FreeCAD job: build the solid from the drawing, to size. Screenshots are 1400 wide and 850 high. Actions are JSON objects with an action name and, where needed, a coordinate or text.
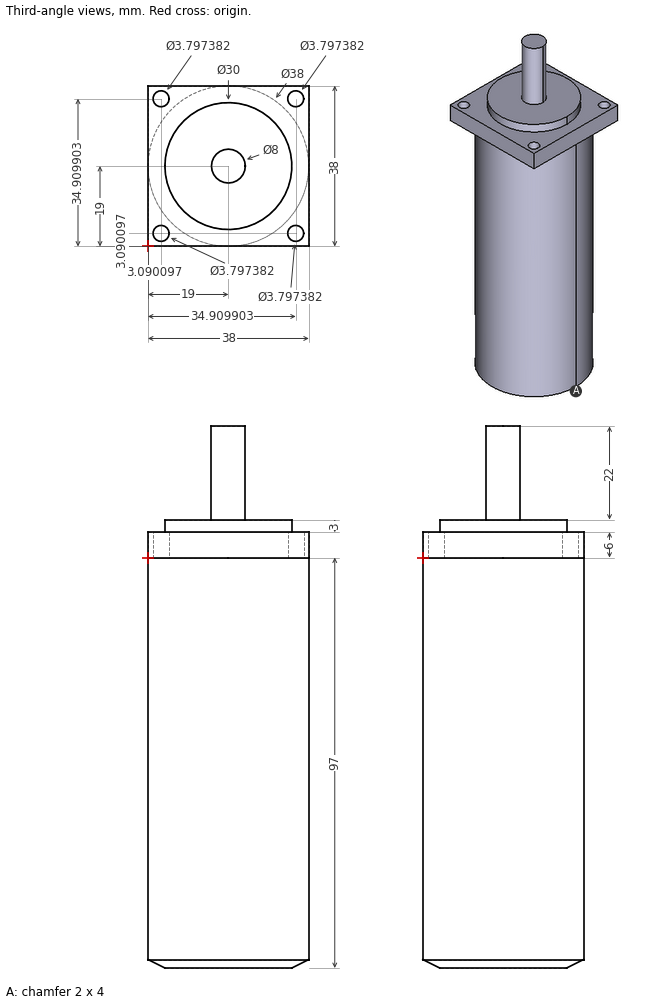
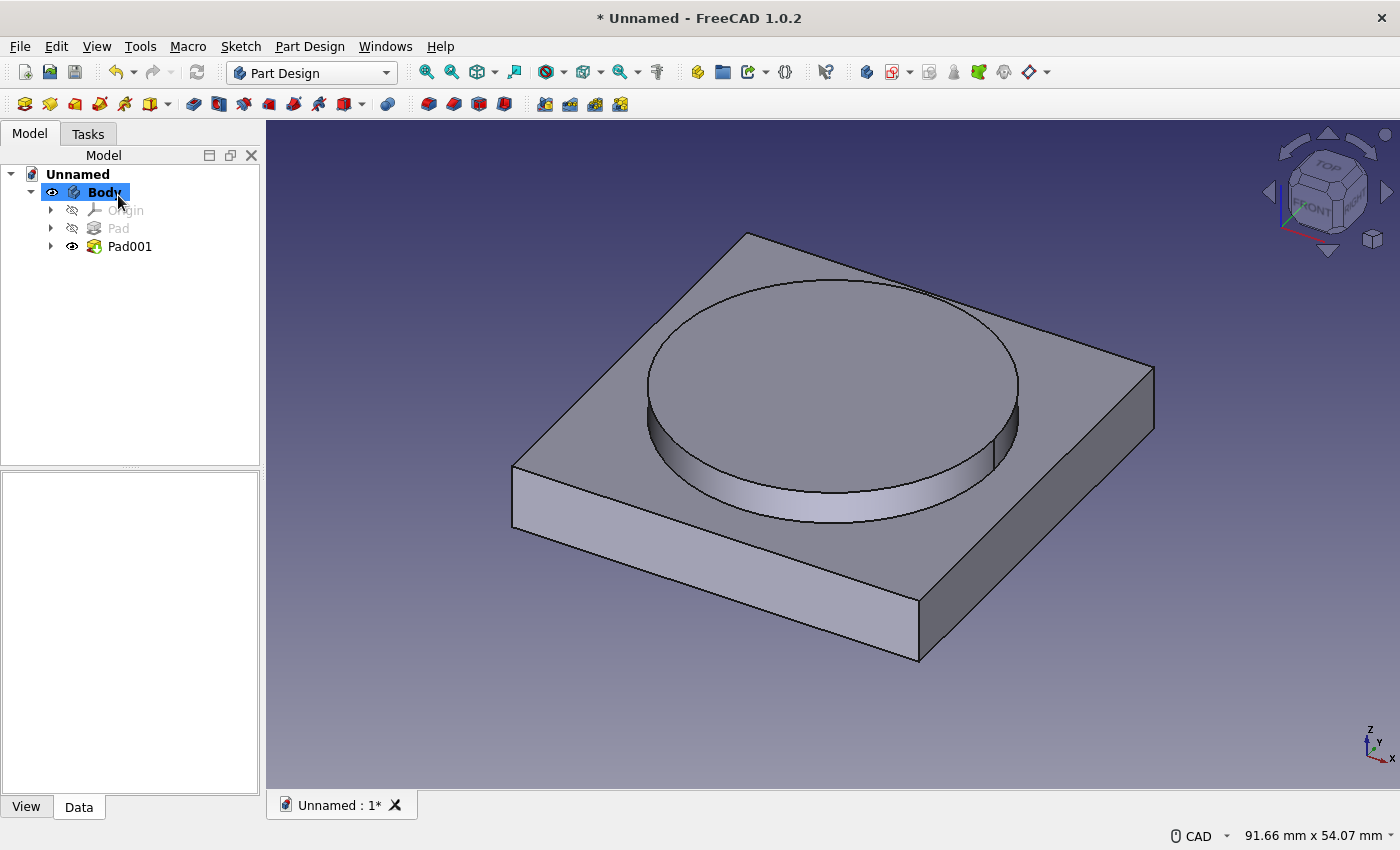
{"action": "left_click", "coordinate": [833, 385]}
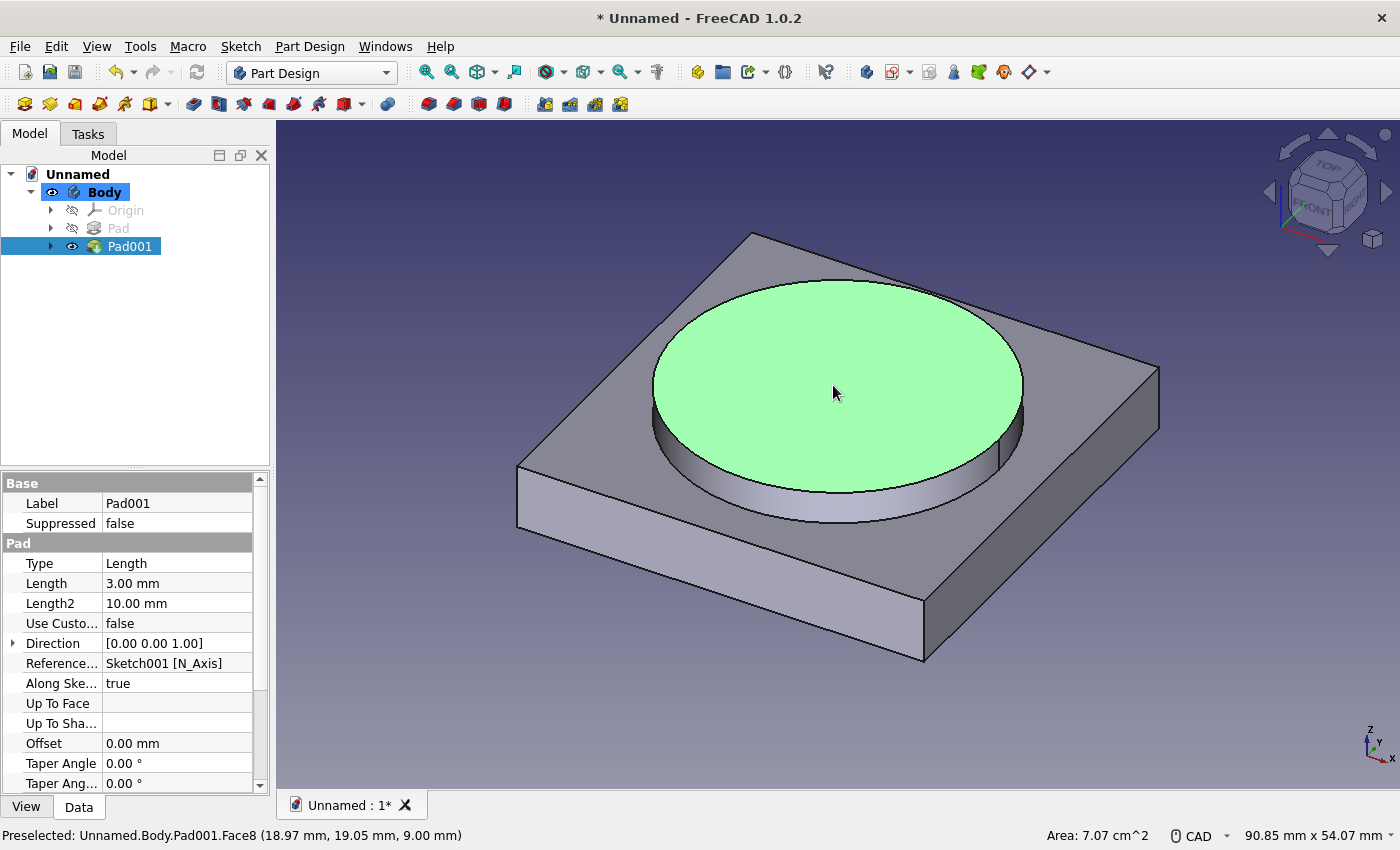
{"action": "left_click", "coordinate": [892, 72]}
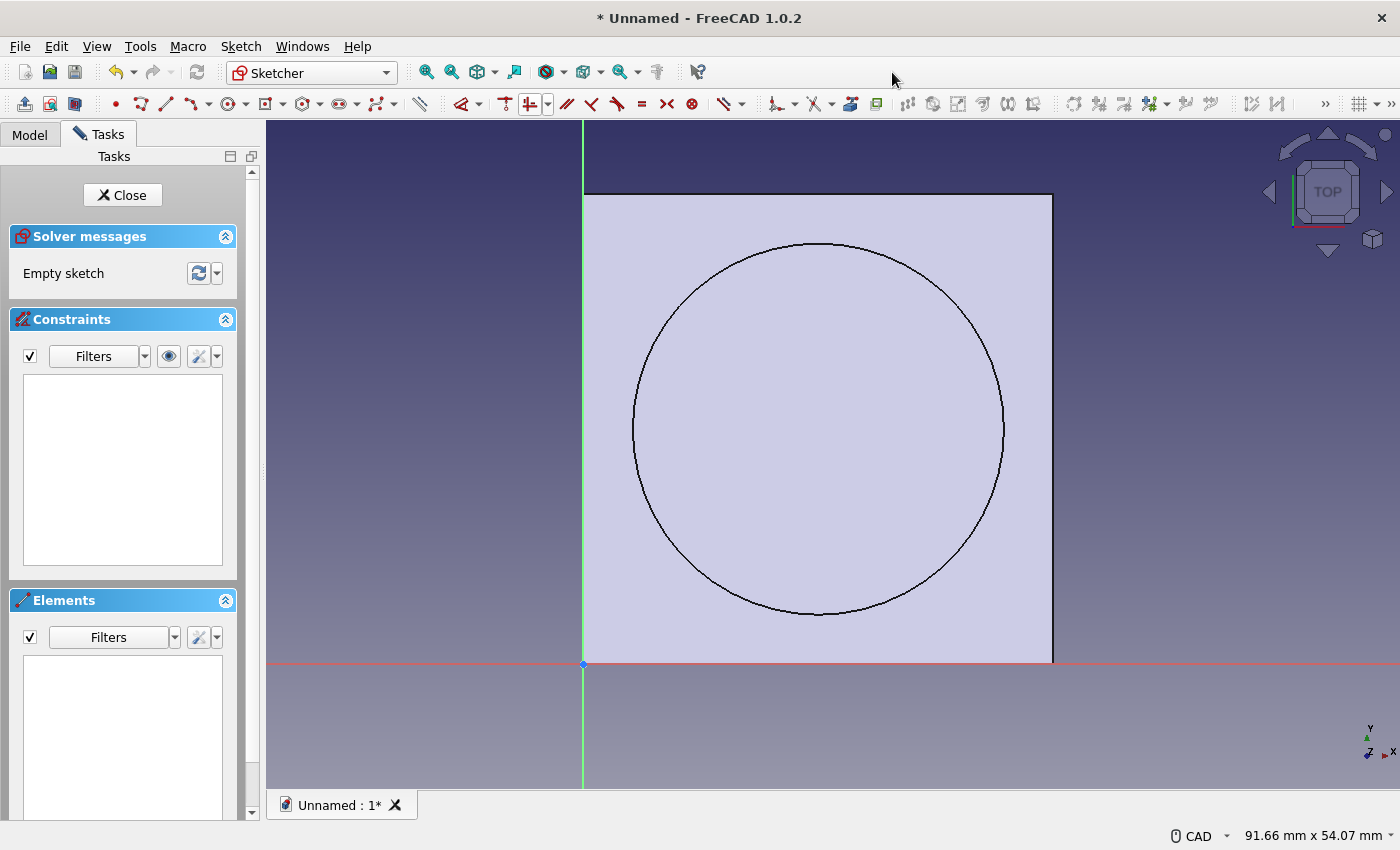
{"action": "scroll", "coordinate": [836, 421], "scroll_direction": "up", "scroll_amount": 7}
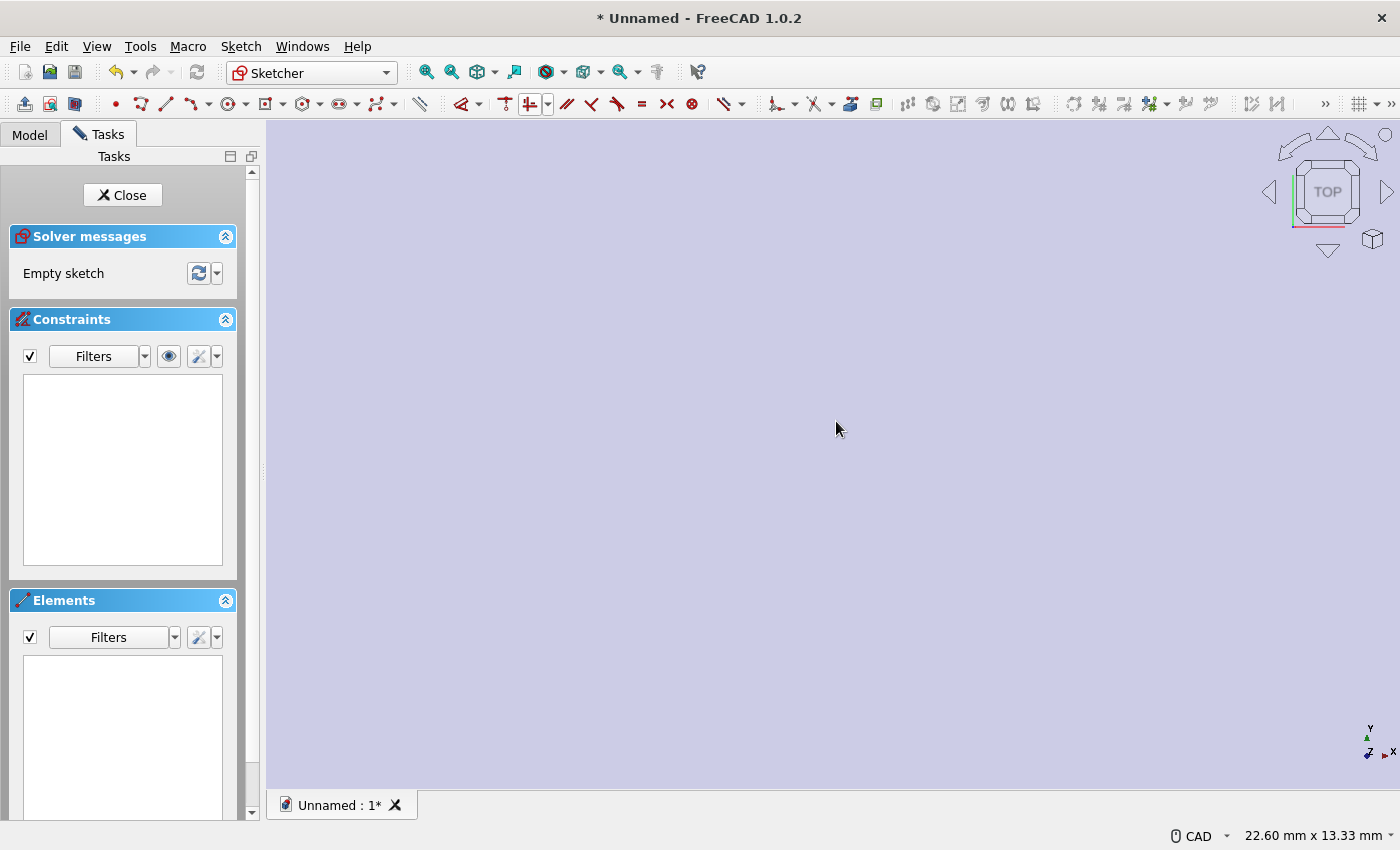
{"action": "left_click", "coordinate": [228, 104]}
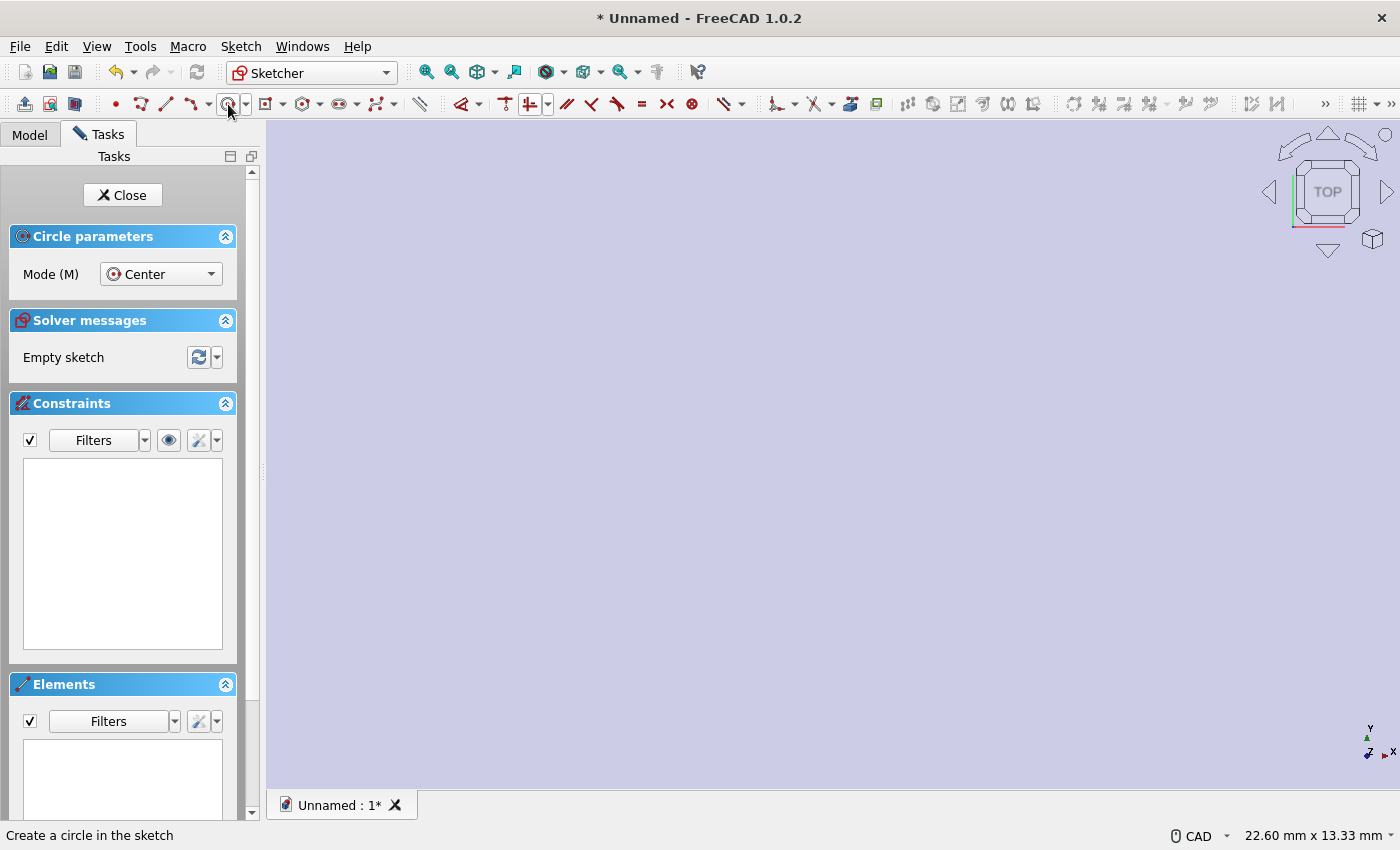
{"action": "left_click", "coordinate": [763, 453]}
{"action": "mouse_move", "coordinate": [905, 311]}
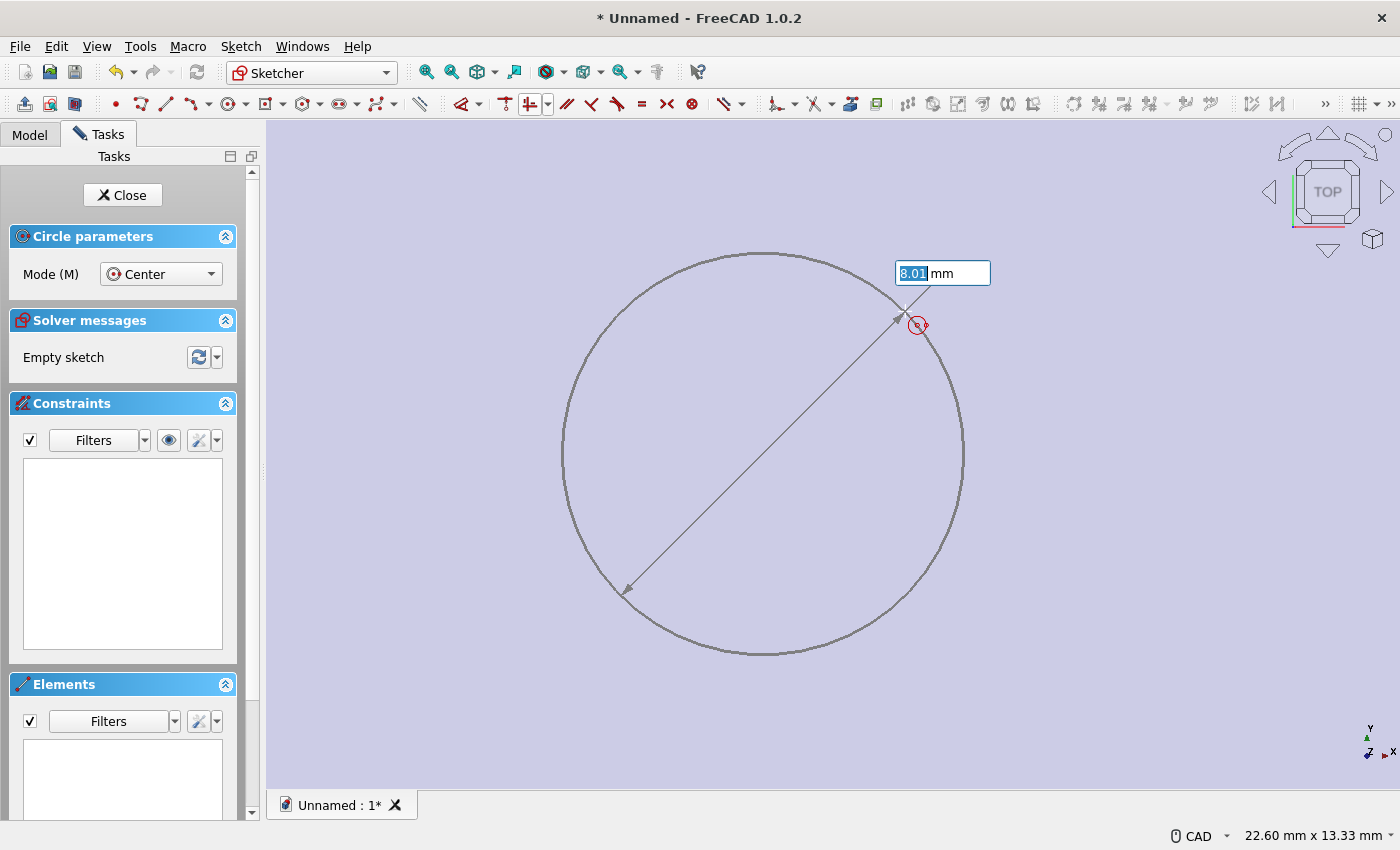
{"action": "type", "text": "8"}
{"action": "key", "text": "Return"}
{"action": "key", "text": "Escape"}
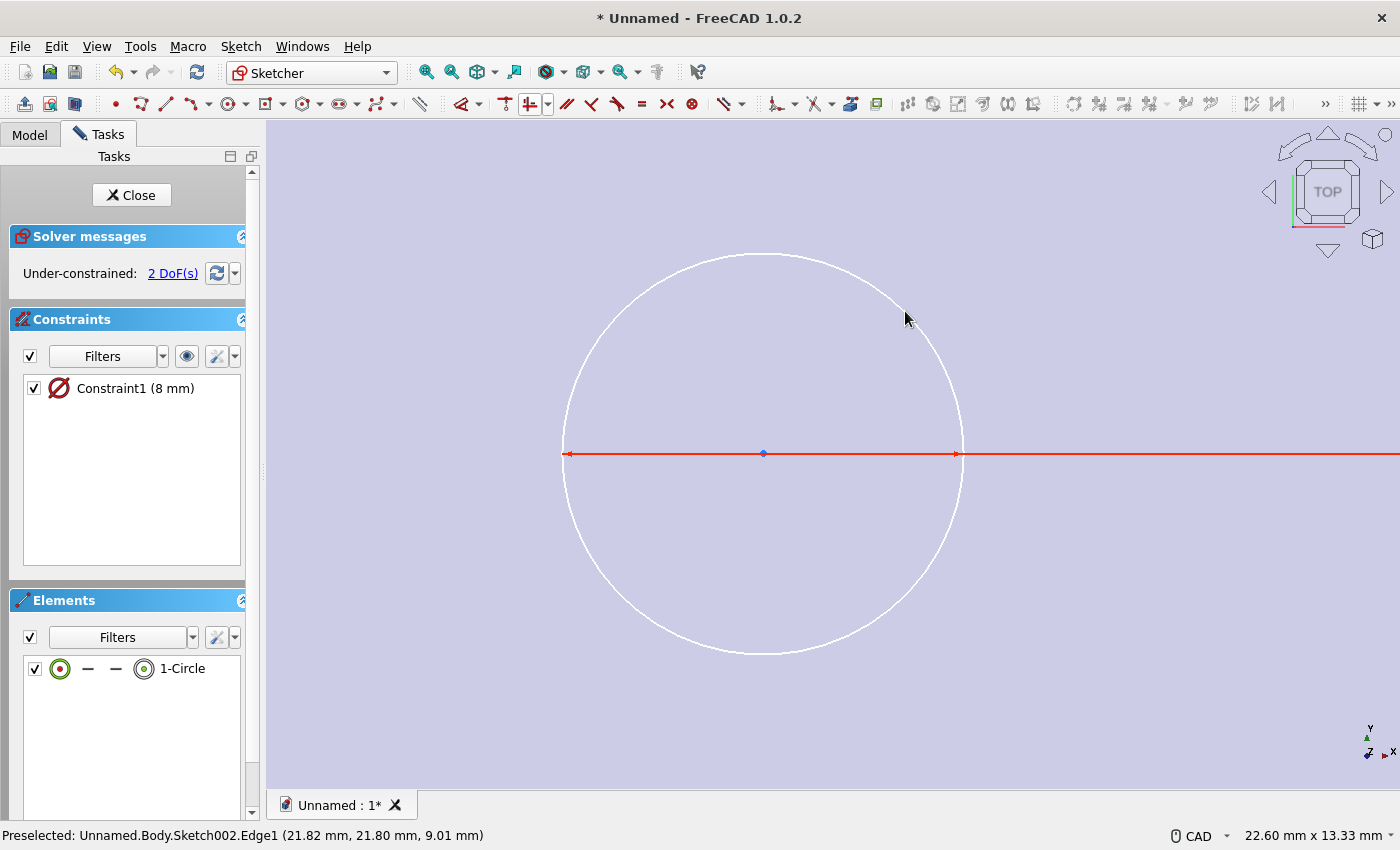
{"action": "key", "text": "d"}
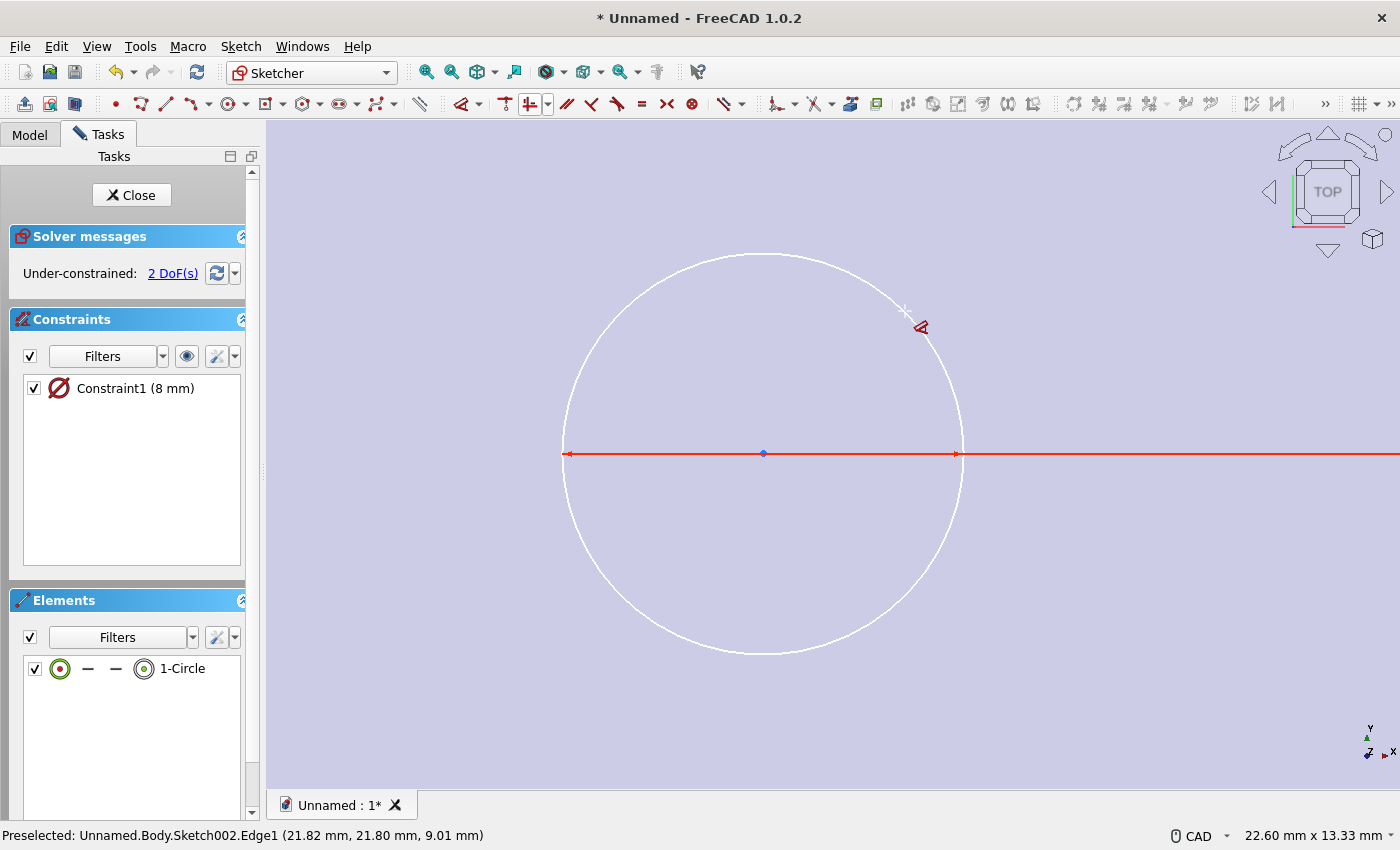
{"action": "left_click", "coordinate": [763, 454]}
{"action": "left_click", "coordinate": [528, 420]}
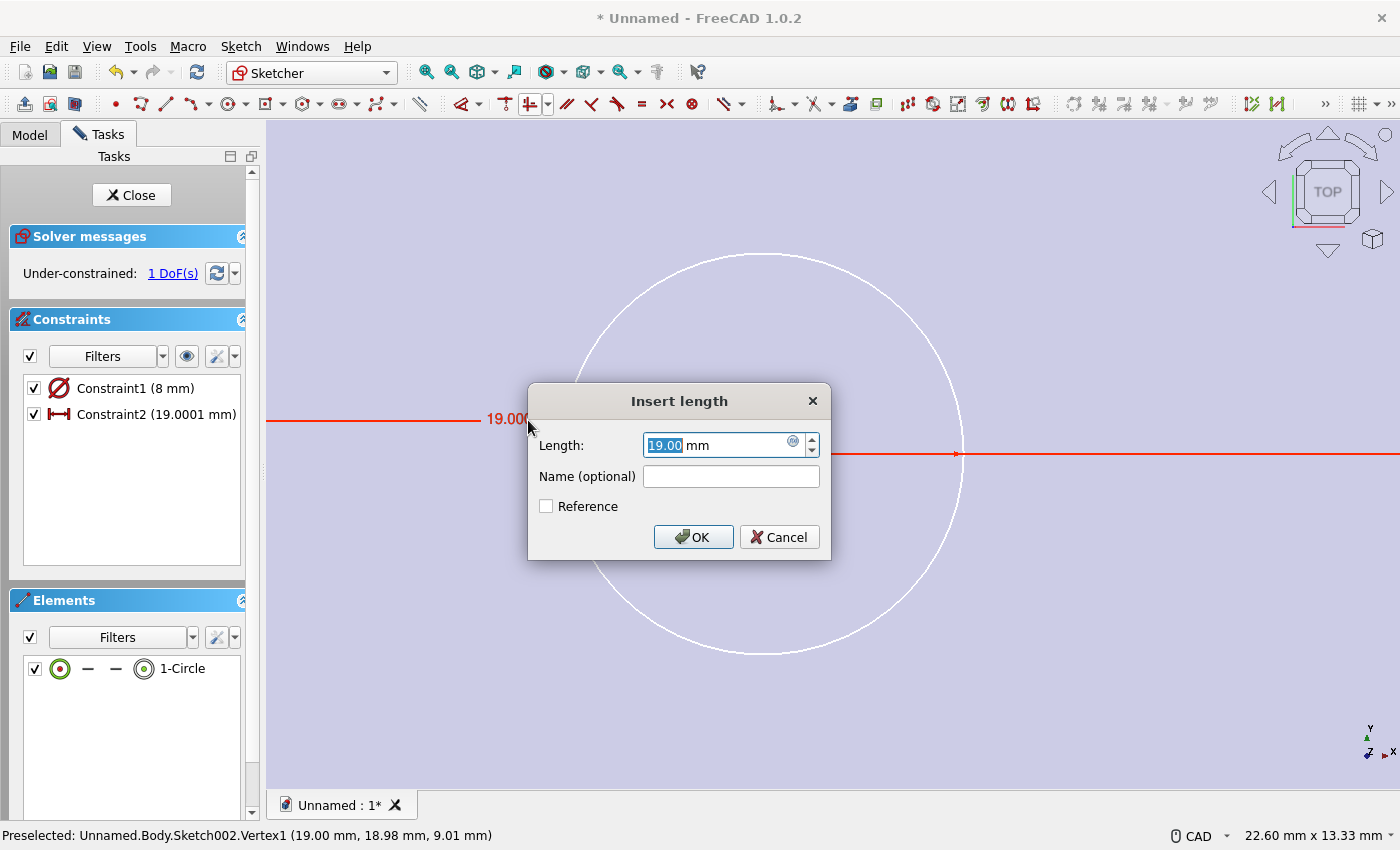
{"action": "type", "text": "19"}
{"action": "key", "text": "Return"}